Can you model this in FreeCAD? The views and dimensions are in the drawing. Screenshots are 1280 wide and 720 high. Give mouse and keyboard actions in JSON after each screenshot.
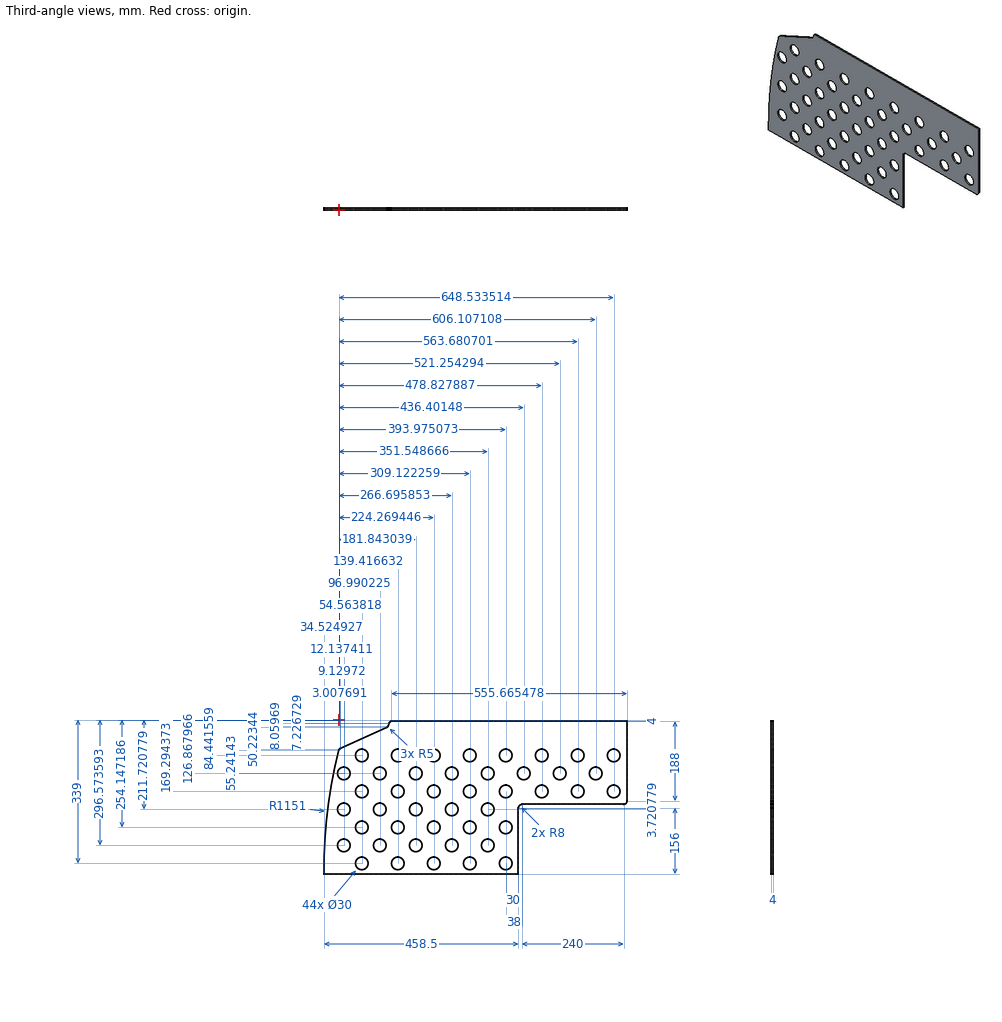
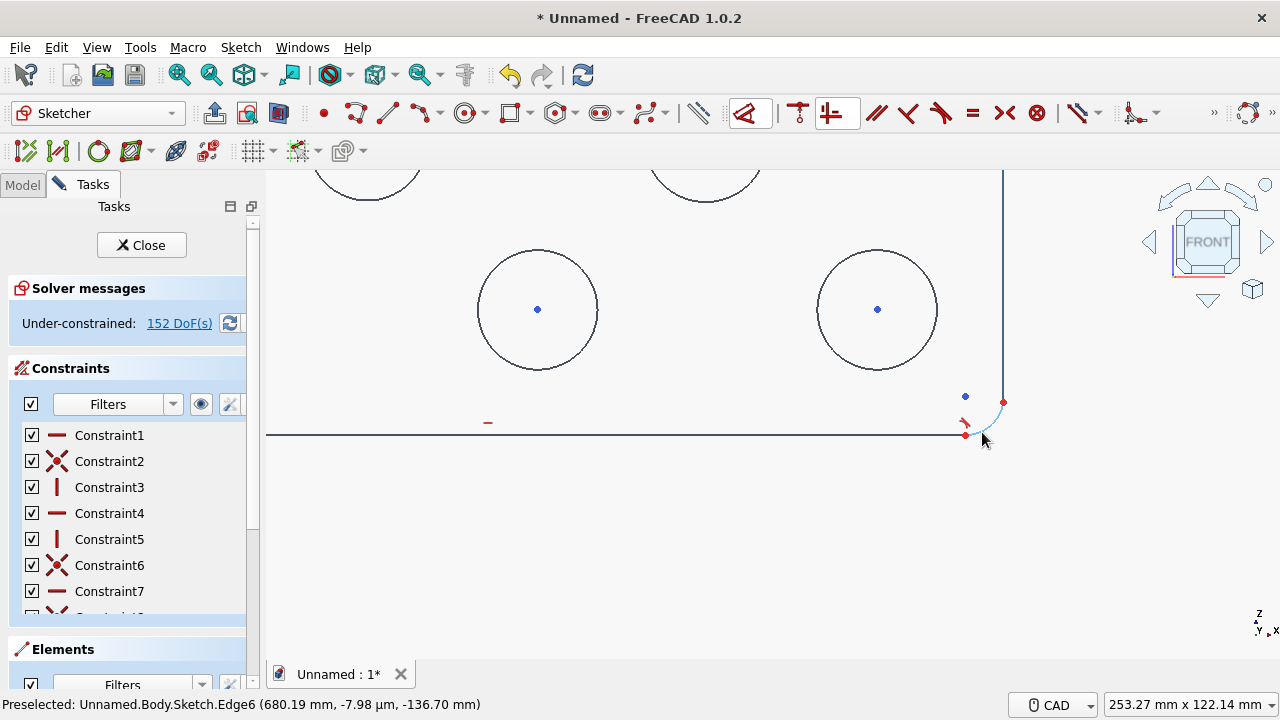
{"action": "left_click", "coordinate": [981, 432]}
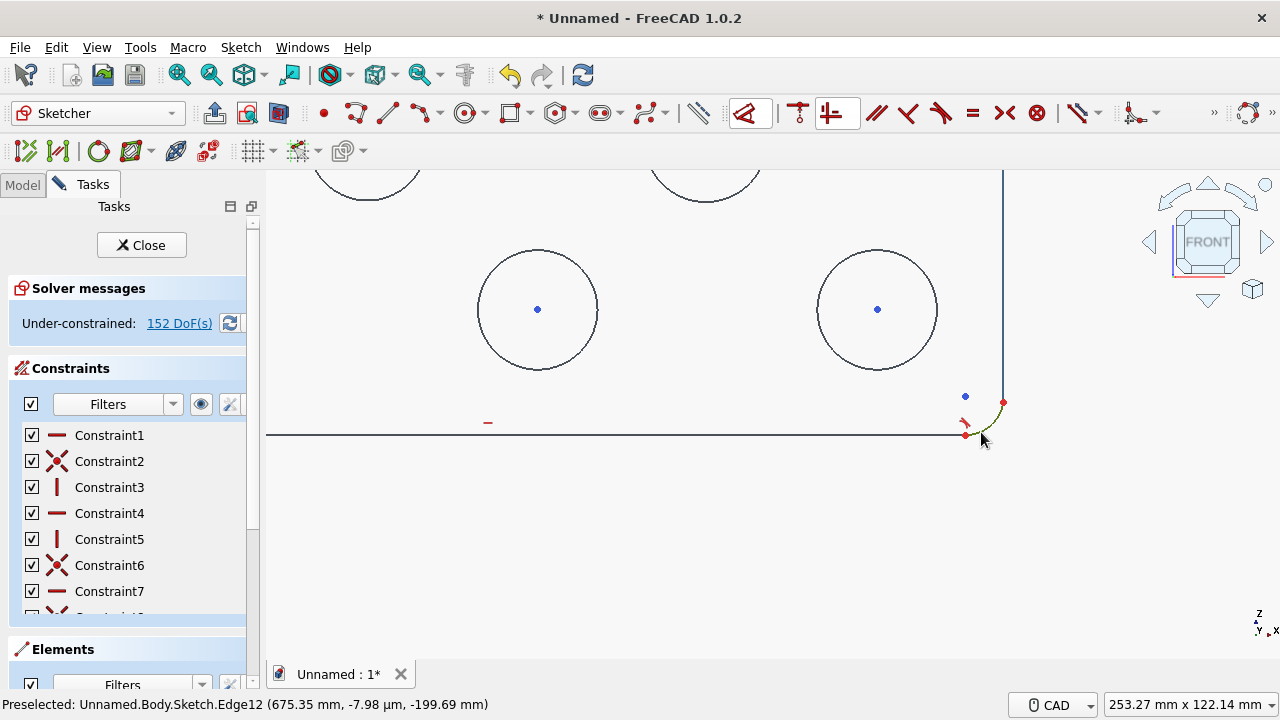
{"action": "key", "text": "t"}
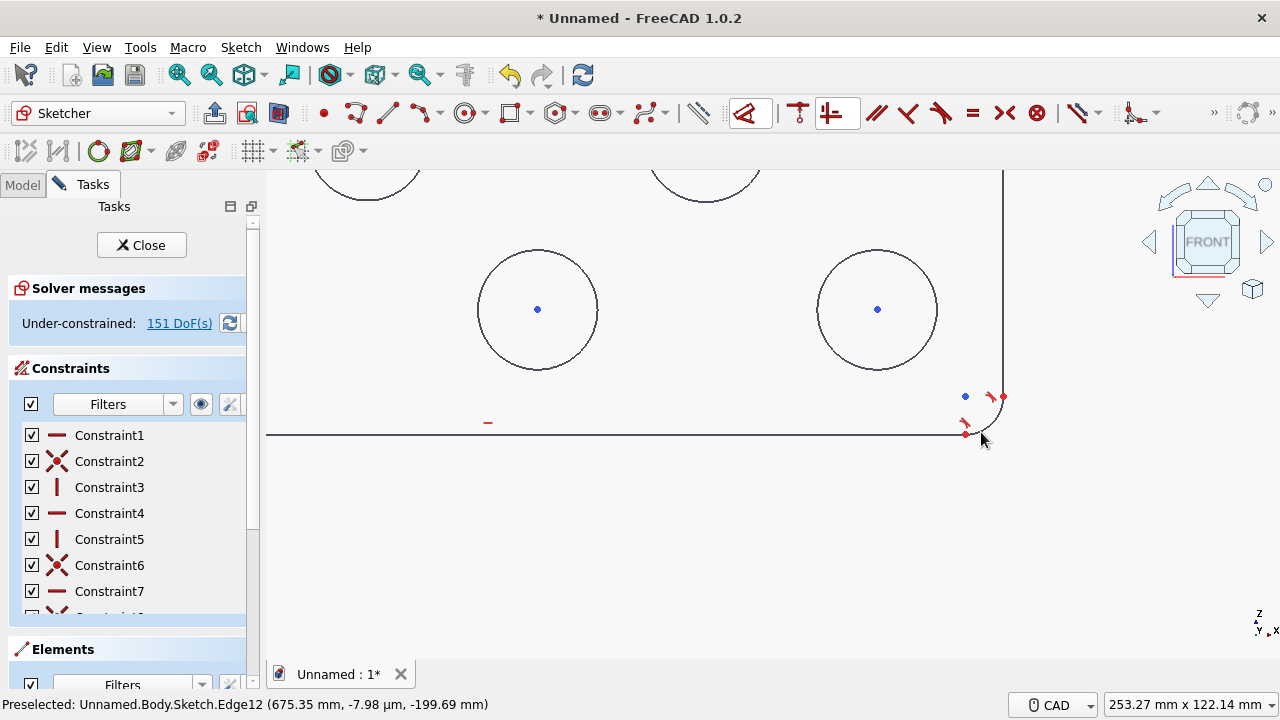
{"action": "scroll", "coordinate": [991, 428], "scroll_direction": "down", "scroll_amount": 8}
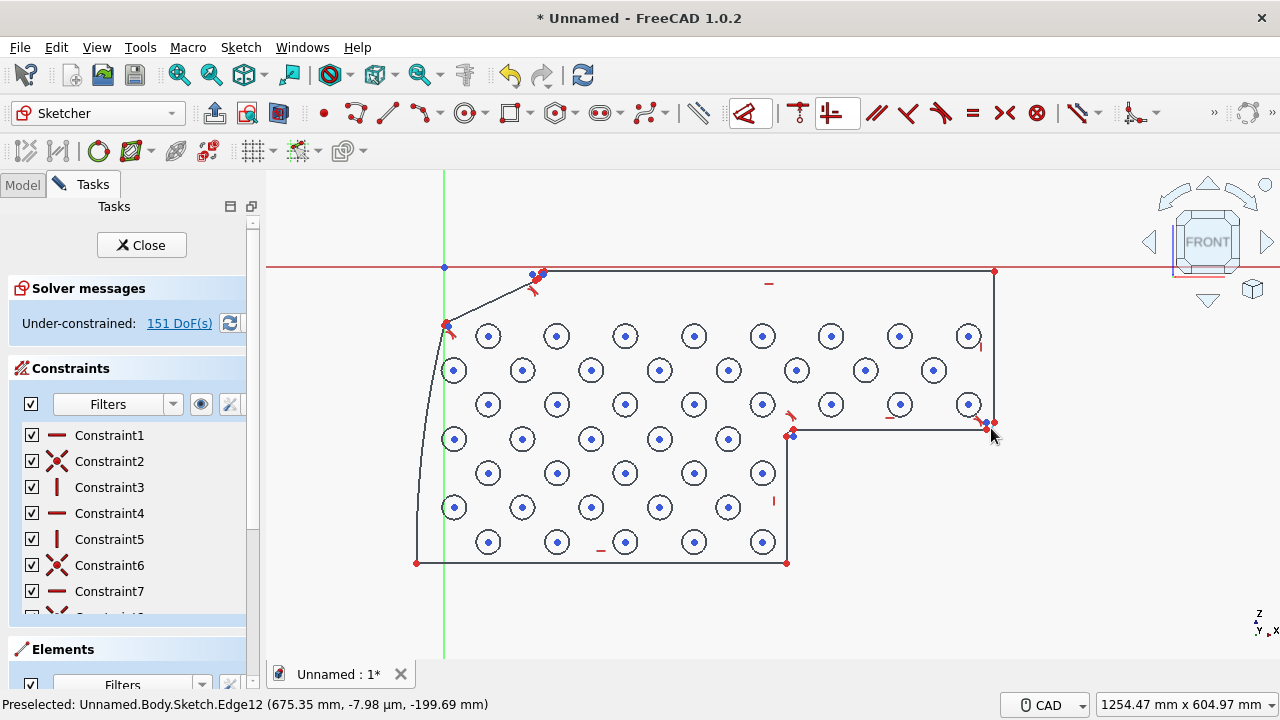
{"action": "scroll", "coordinate": [859, 271], "scroll_direction": "up", "scroll_amount": 7}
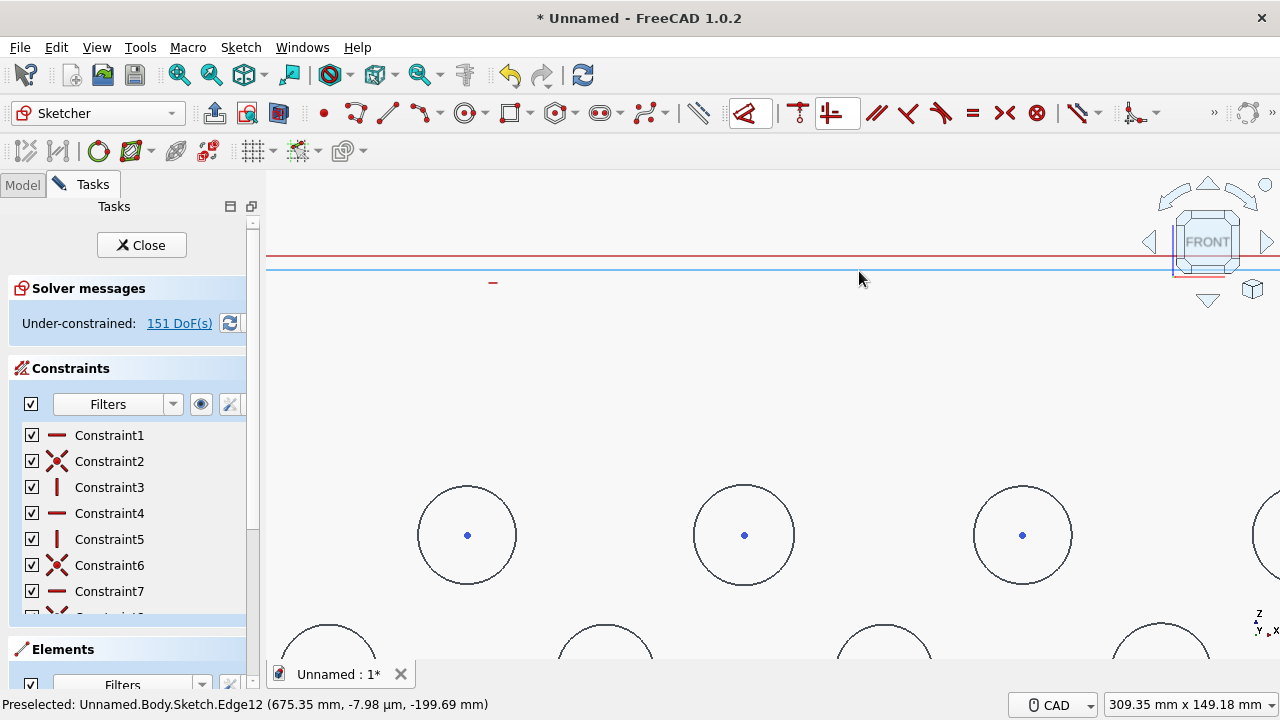
{"action": "left_click", "coordinate": [858, 270]}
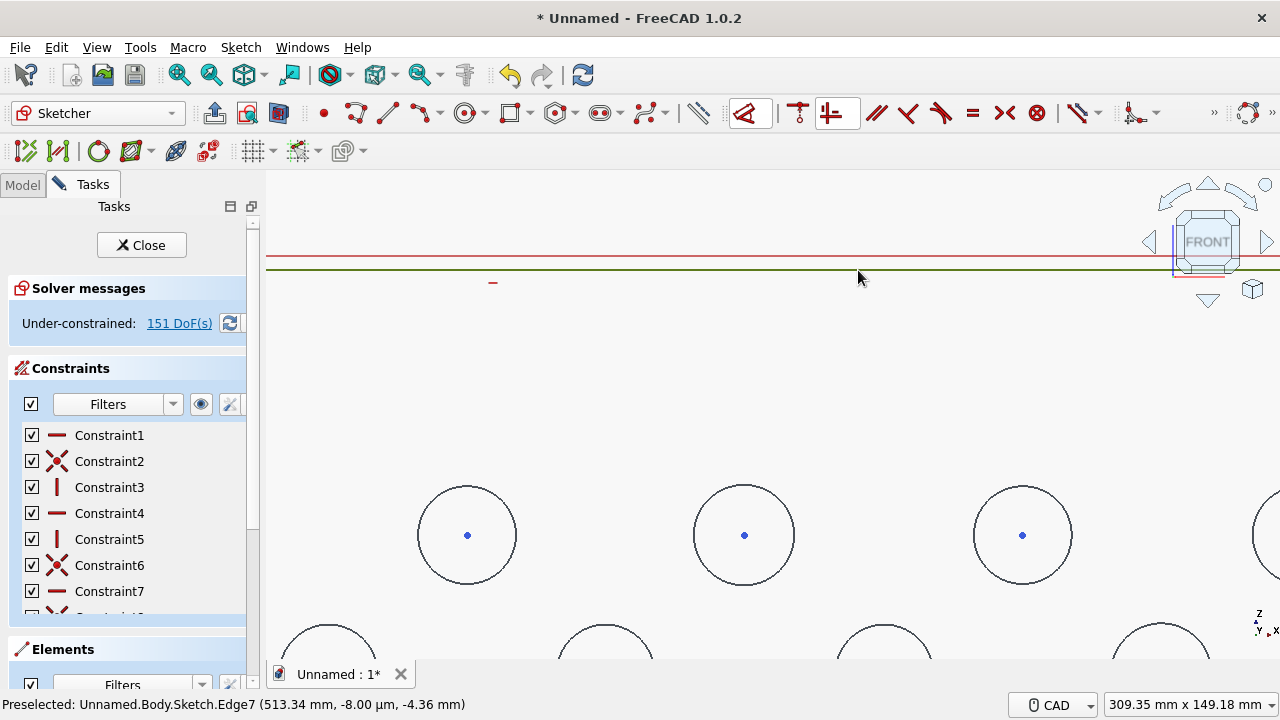
{"action": "scroll", "coordinate": [859, 271], "scroll_direction": "down", "scroll_amount": 7}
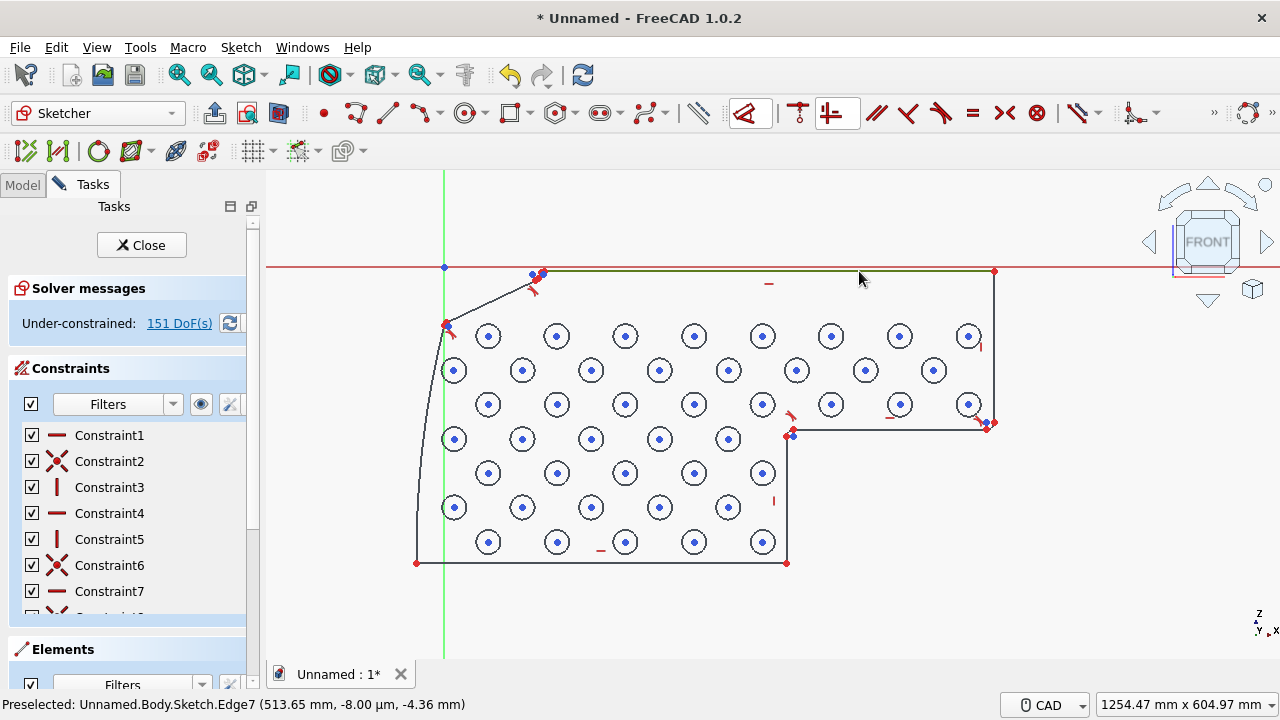
{"action": "scroll", "coordinate": [543, 271], "scroll_direction": "up", "scroll_amount": 10}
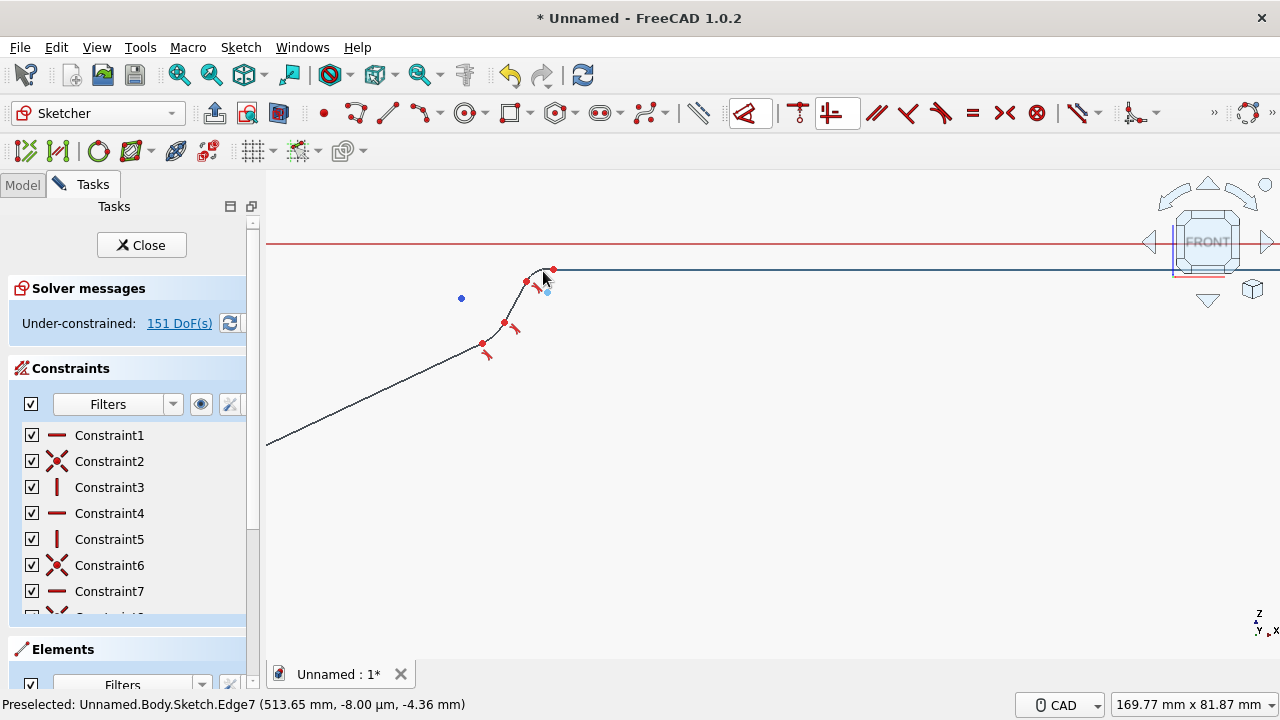
{"action": "left_click", "coordinate": [538, 271]}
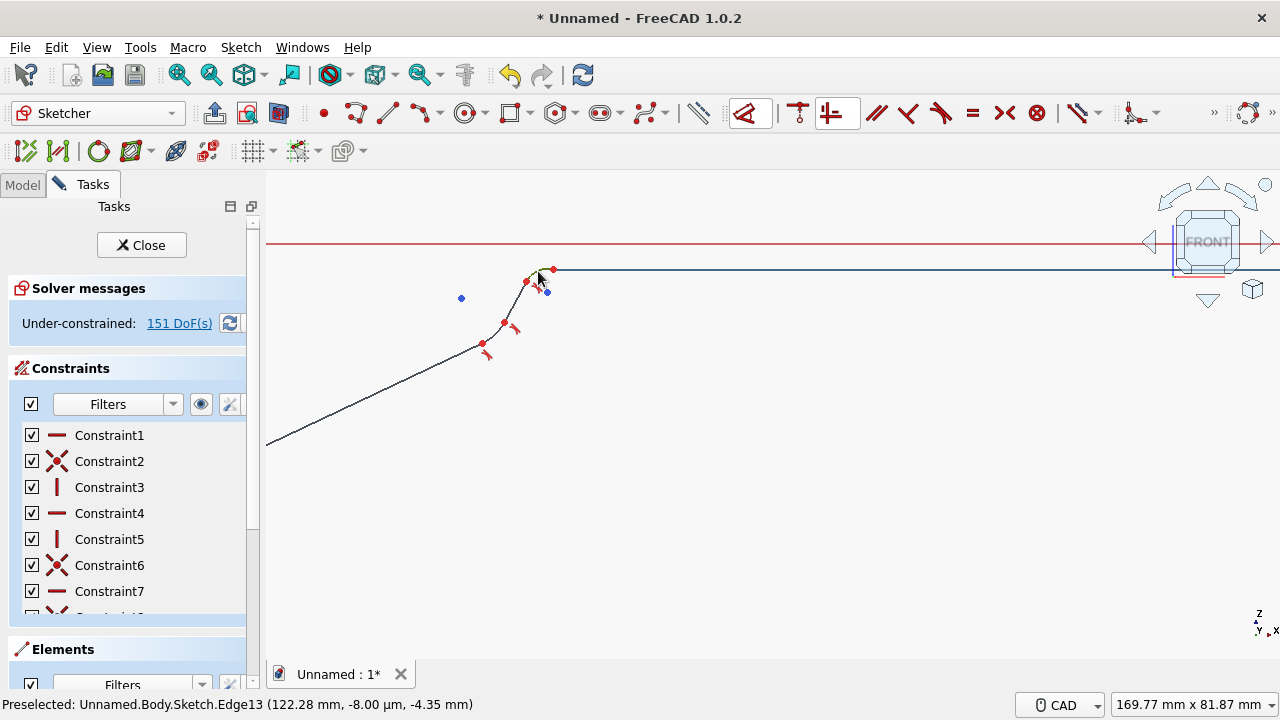
{"action": "key", "text": "t"}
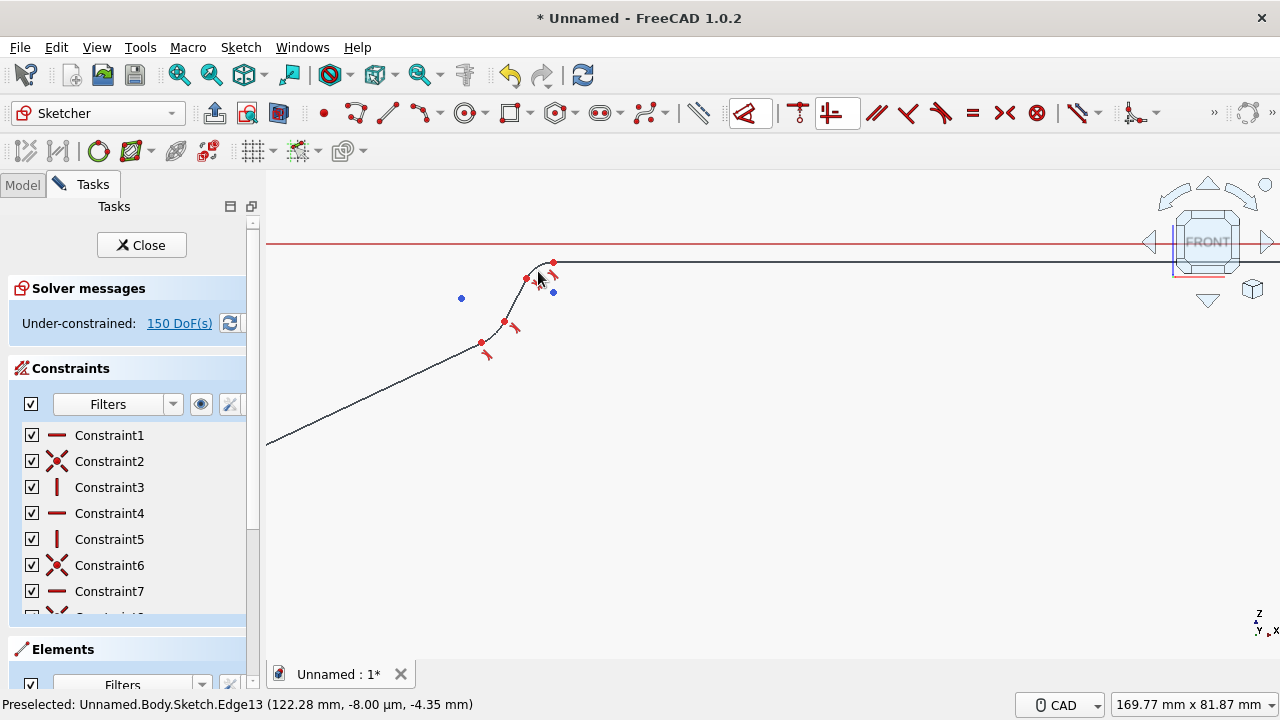
{"action": "scroll", "coordinate": [543, 271], "scroll_direction": "down", "scroll_amount": 10}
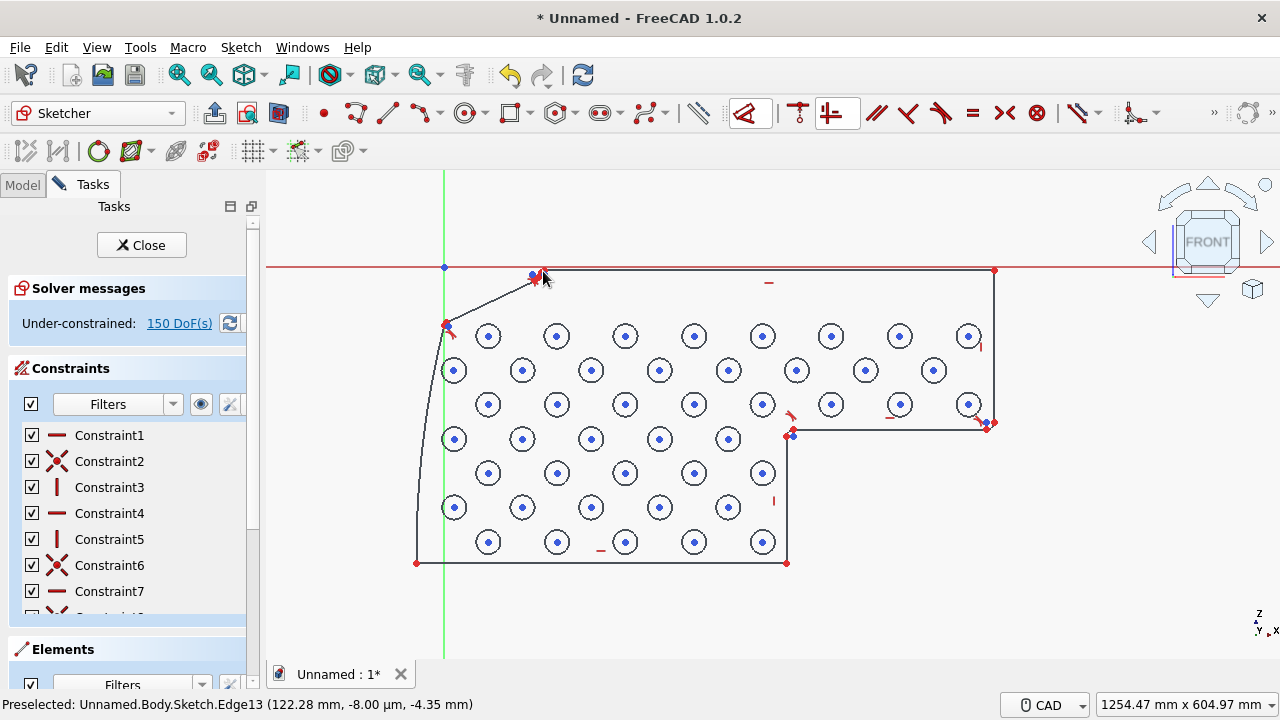
{"action": "scroll", "coordinate": [445, 324], "scroll_direction": "up", "scroll_amount": 13}